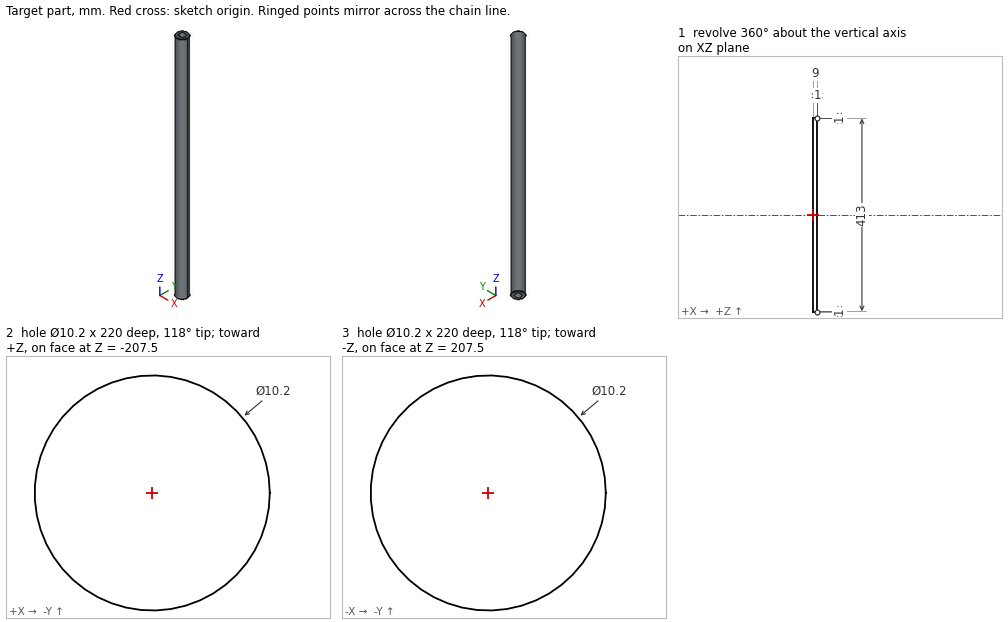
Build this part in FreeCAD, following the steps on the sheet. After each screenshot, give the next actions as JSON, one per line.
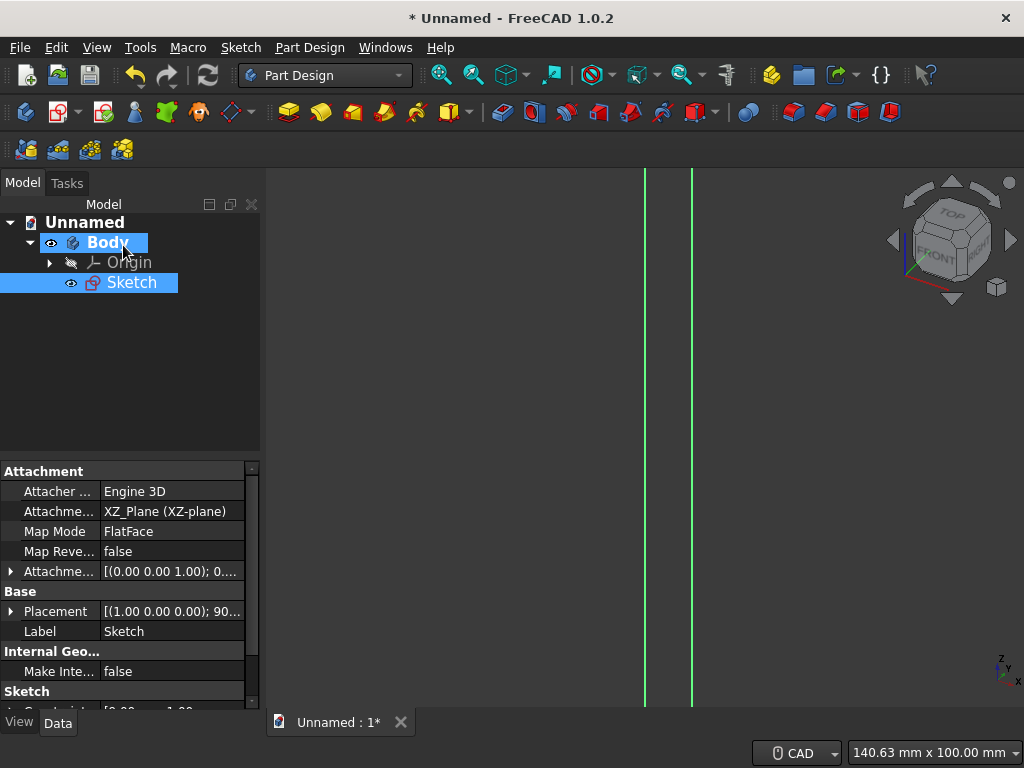
{"action": "left_click", "coordinate": [322, 112]}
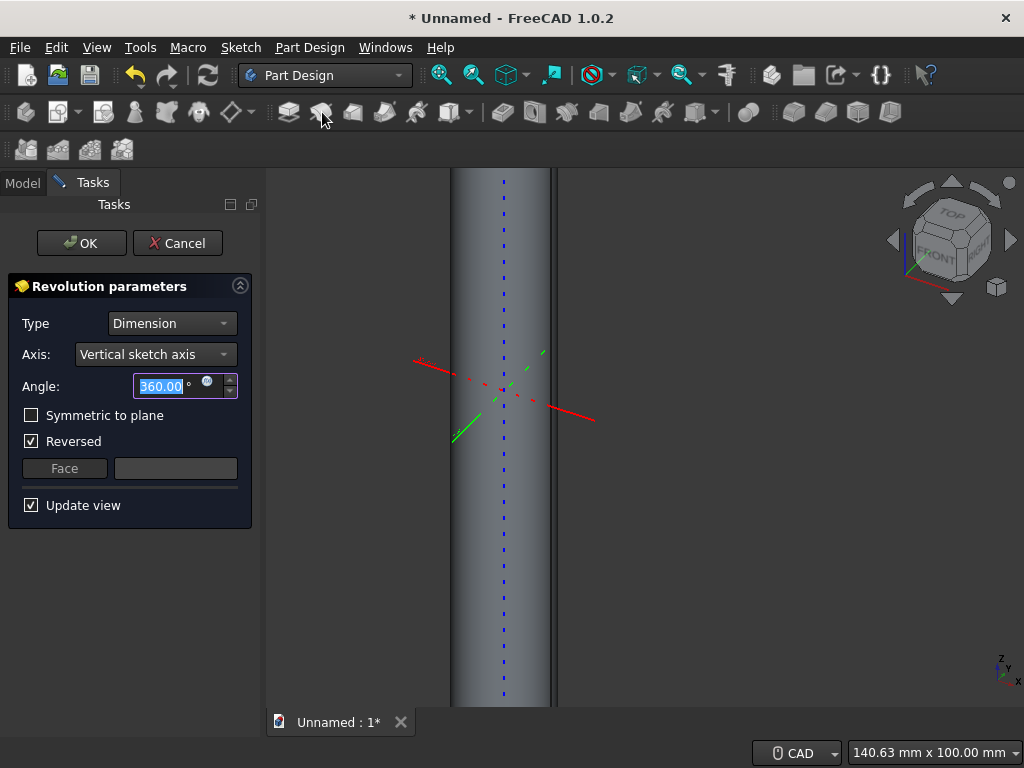
{"action": "left_click", "coordinate": [82, 243]}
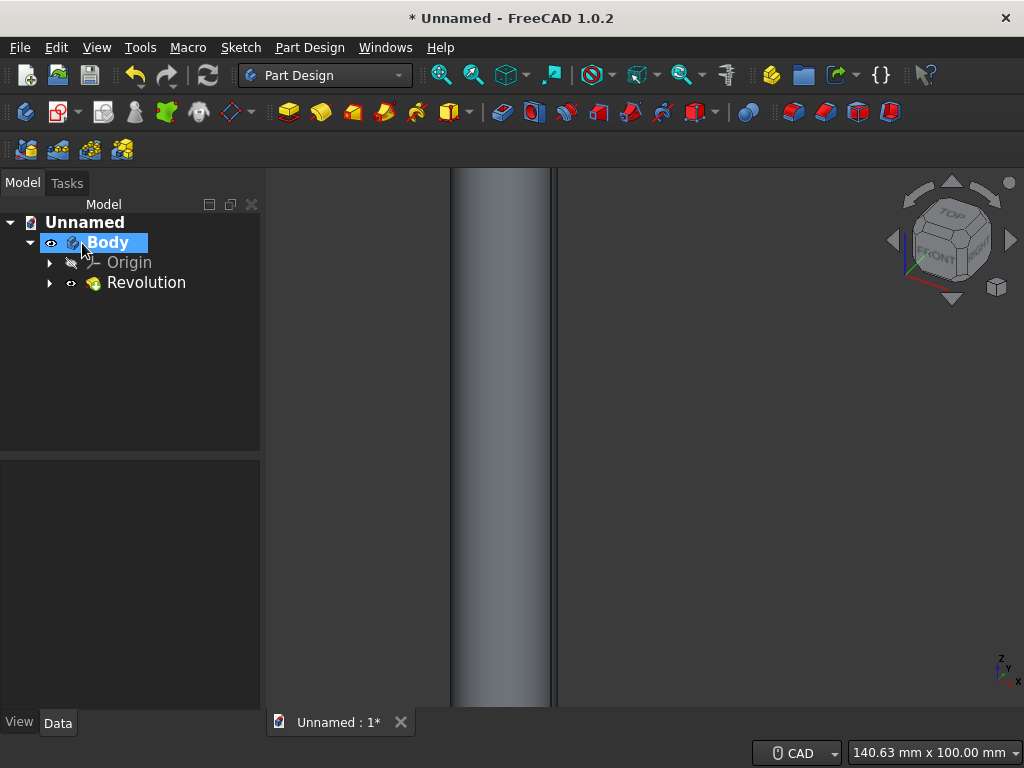
{"action": "left_click", "coordinate": [442, 76]}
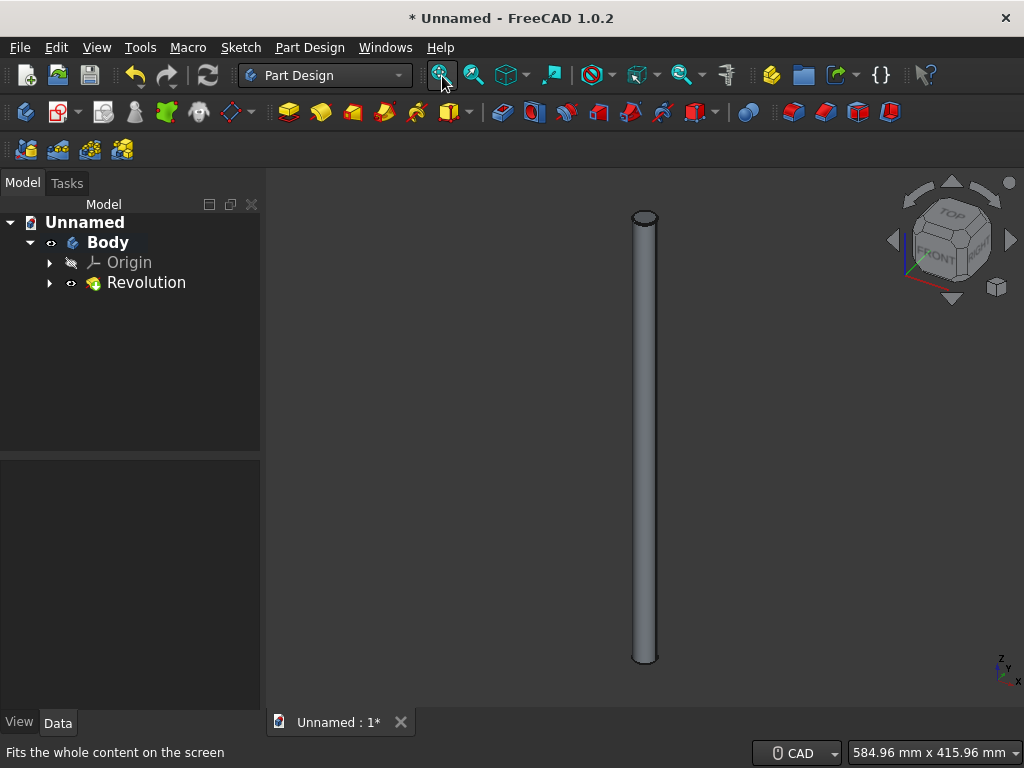
{"action": "key", "text": "5"}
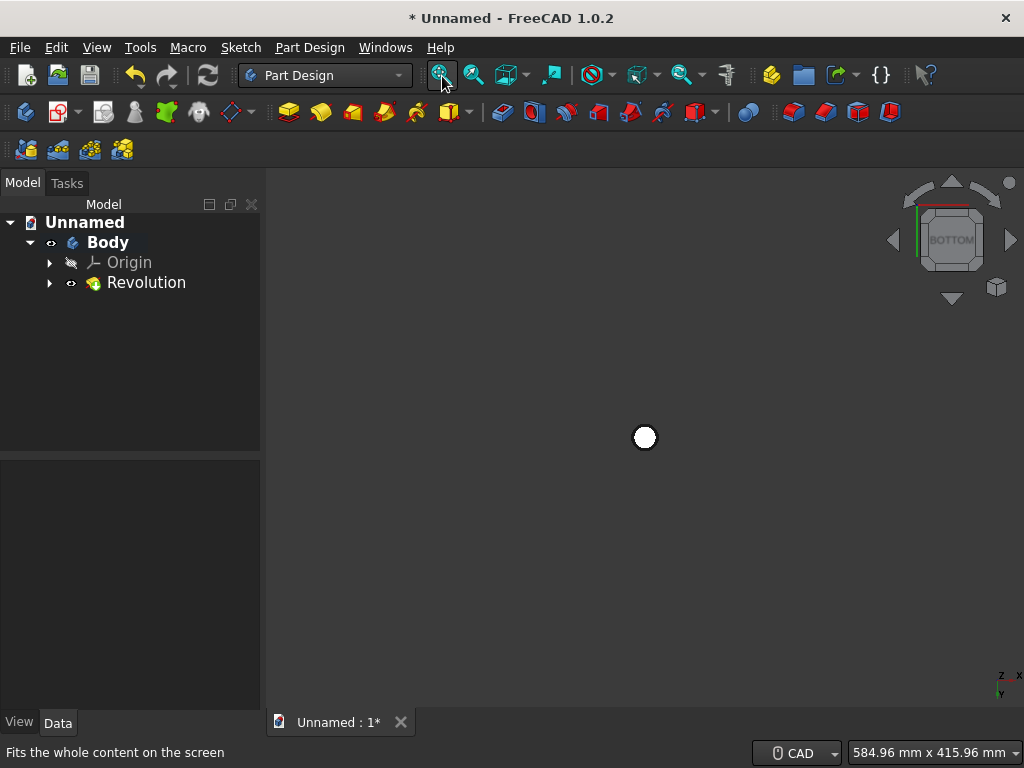
{"action": "left_click", "coordinate": [442, 76]}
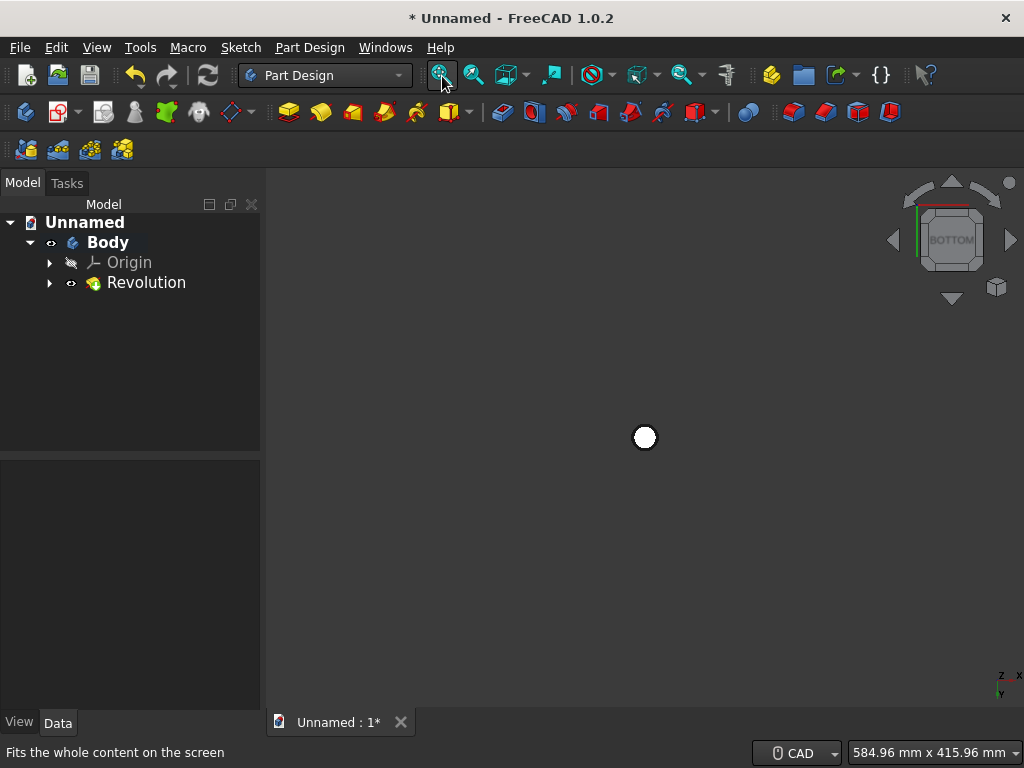
{"action": "left_click", "coordinate": [645, 436]}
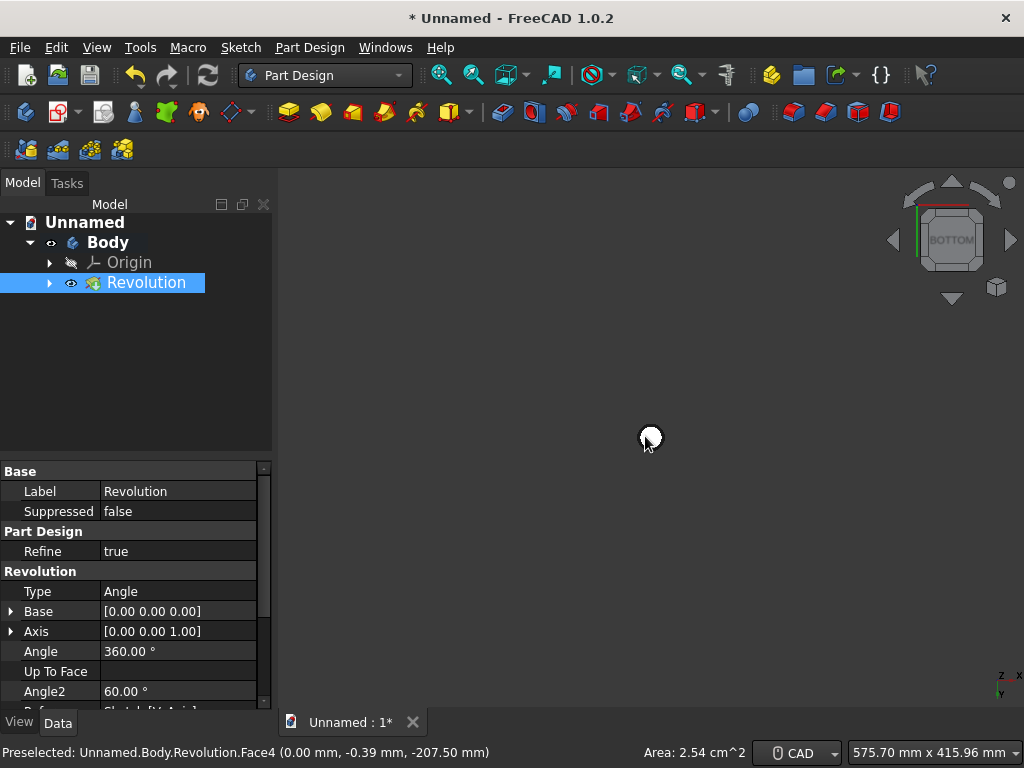
{"action": "left_click", "coordinate": [58, 112]}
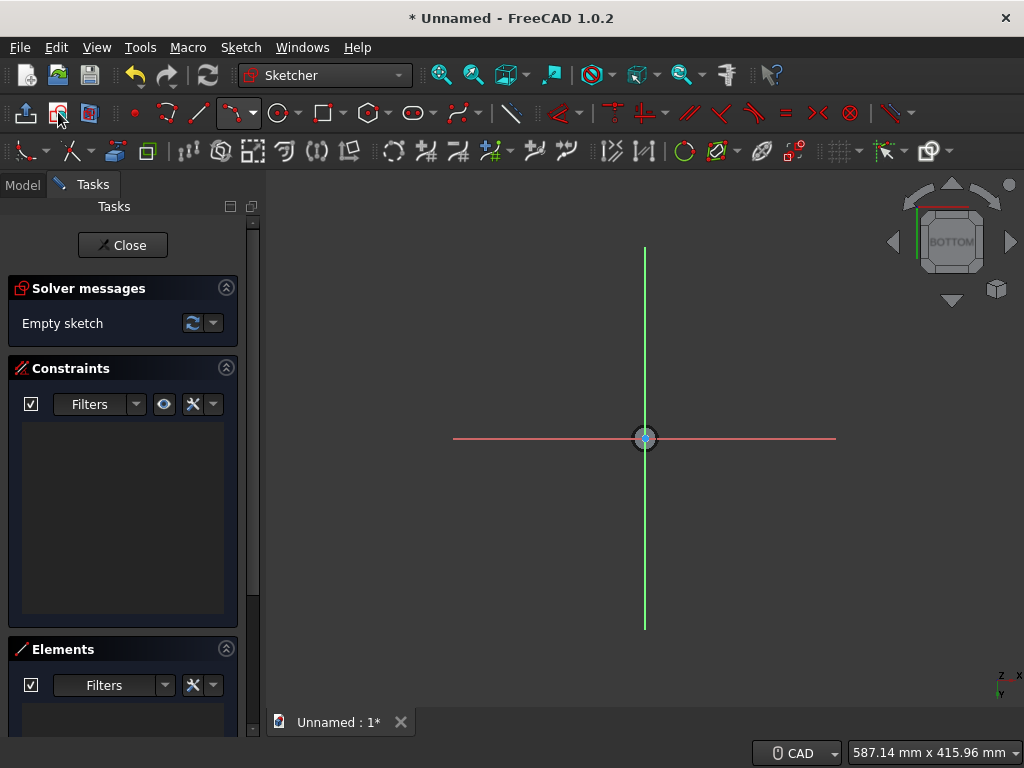
{"action": "scroll", "coordinate": [649, 438], "scroll_direction": "up", "scroll_amount": 15}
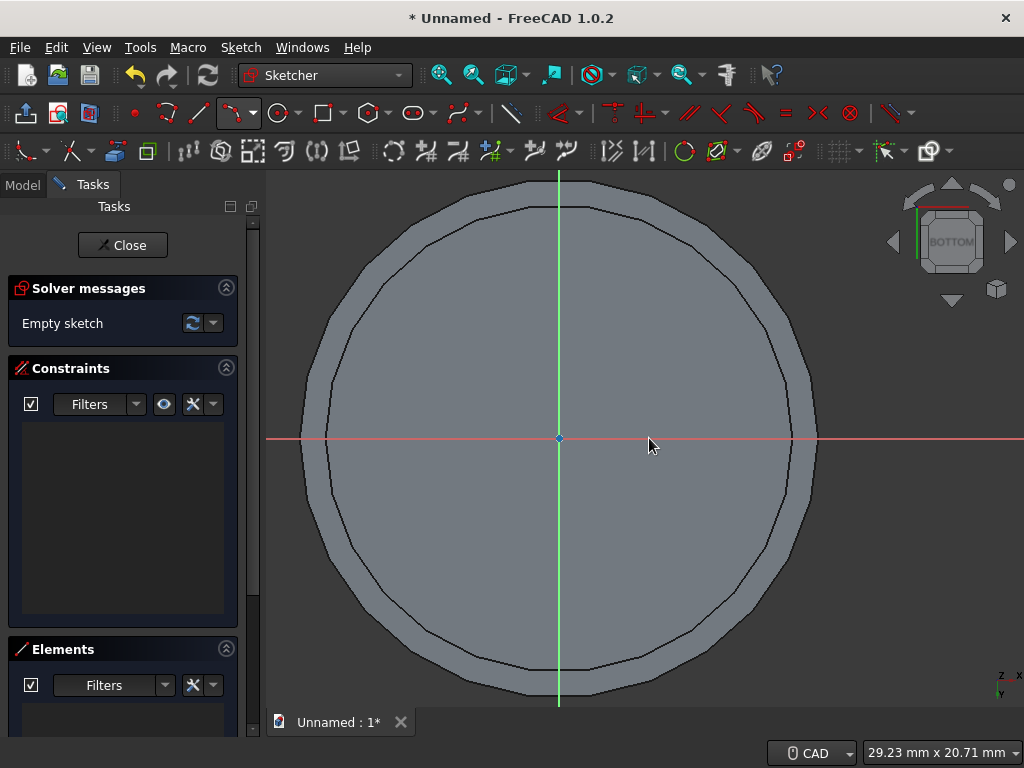
{"action": "left_click", "coordinate": [278, 114]}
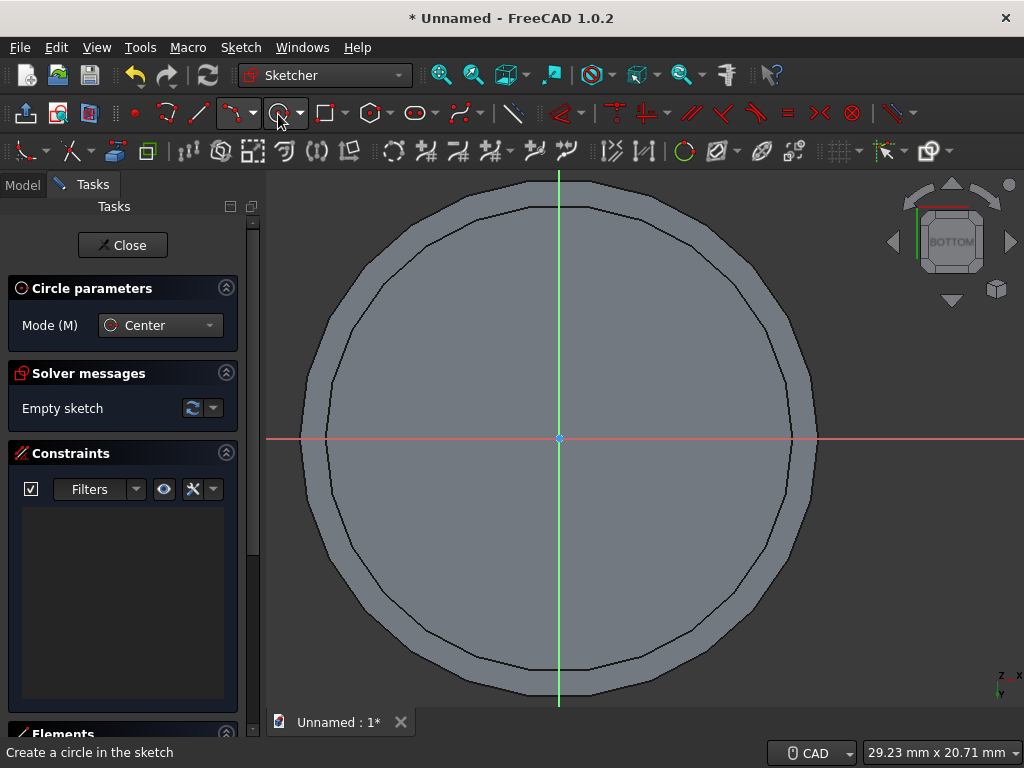
{"action": "left_click", "coordinate": [559, 438]}
{"action": "left_click", "coordinate": [653, 345]}
{"action": "key", "text": "Escape"}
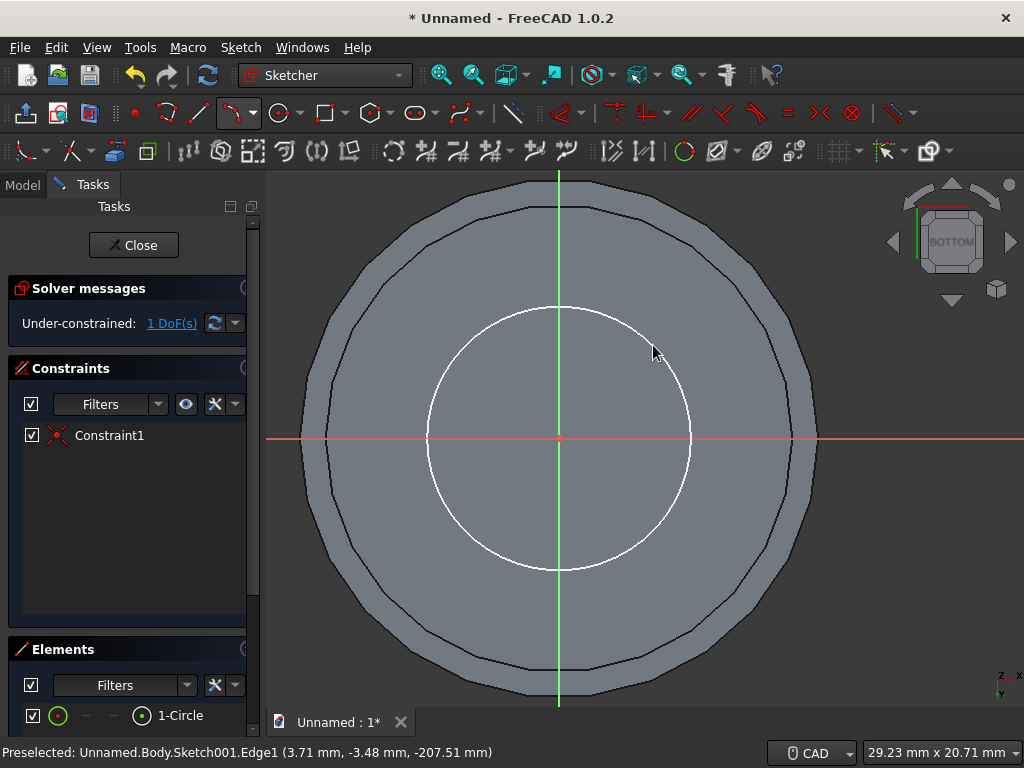
{"action": "key", "text": "d"}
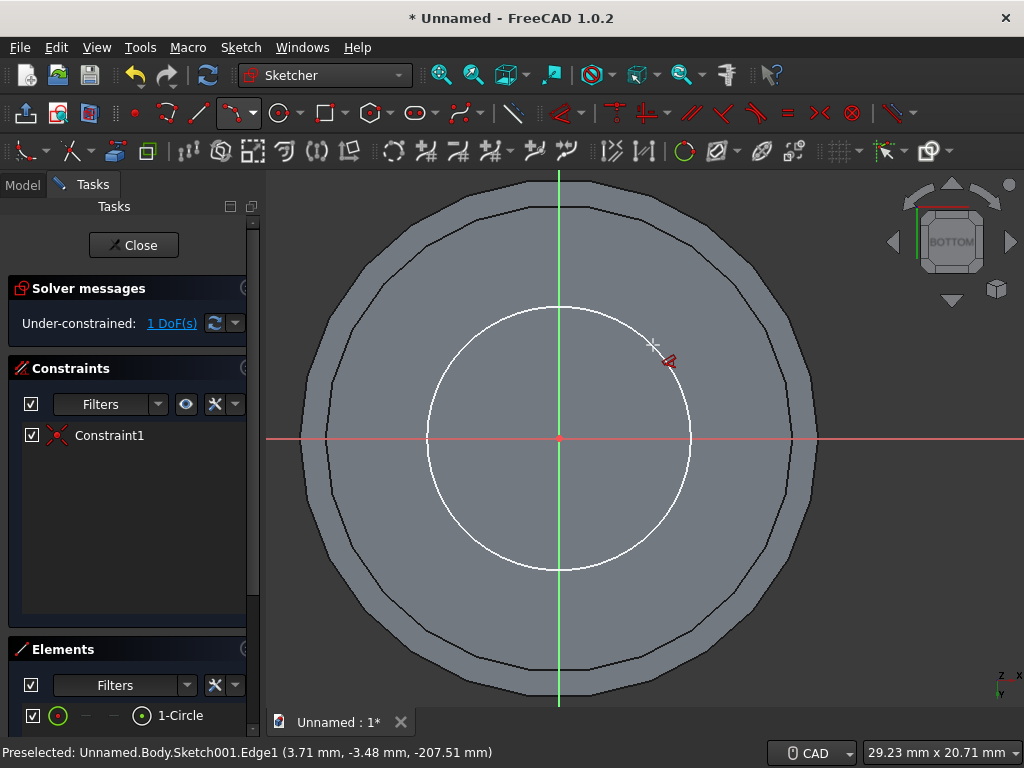
{"action": "left_click", "coordinate": [652, 345]}
{"action": "left_click", "coordinate": [675, 322]}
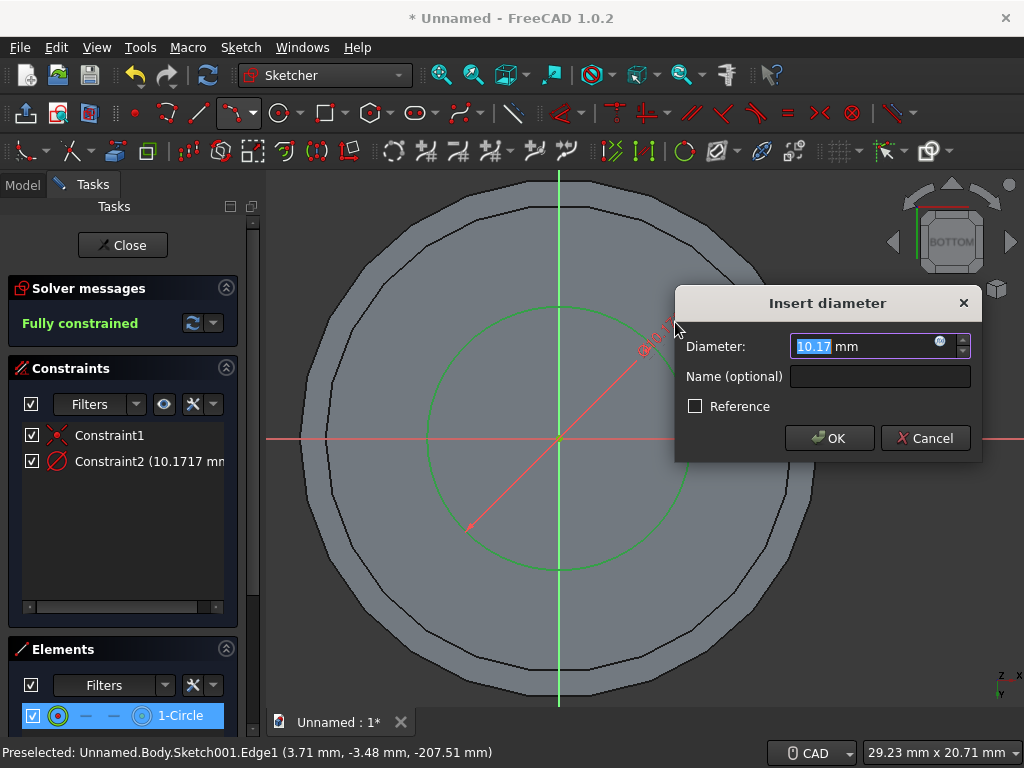
{"action": "type", "text": "10.2"}
{"action": "key", "text": "Return"}
{"action": "key", "text": "Escape"}